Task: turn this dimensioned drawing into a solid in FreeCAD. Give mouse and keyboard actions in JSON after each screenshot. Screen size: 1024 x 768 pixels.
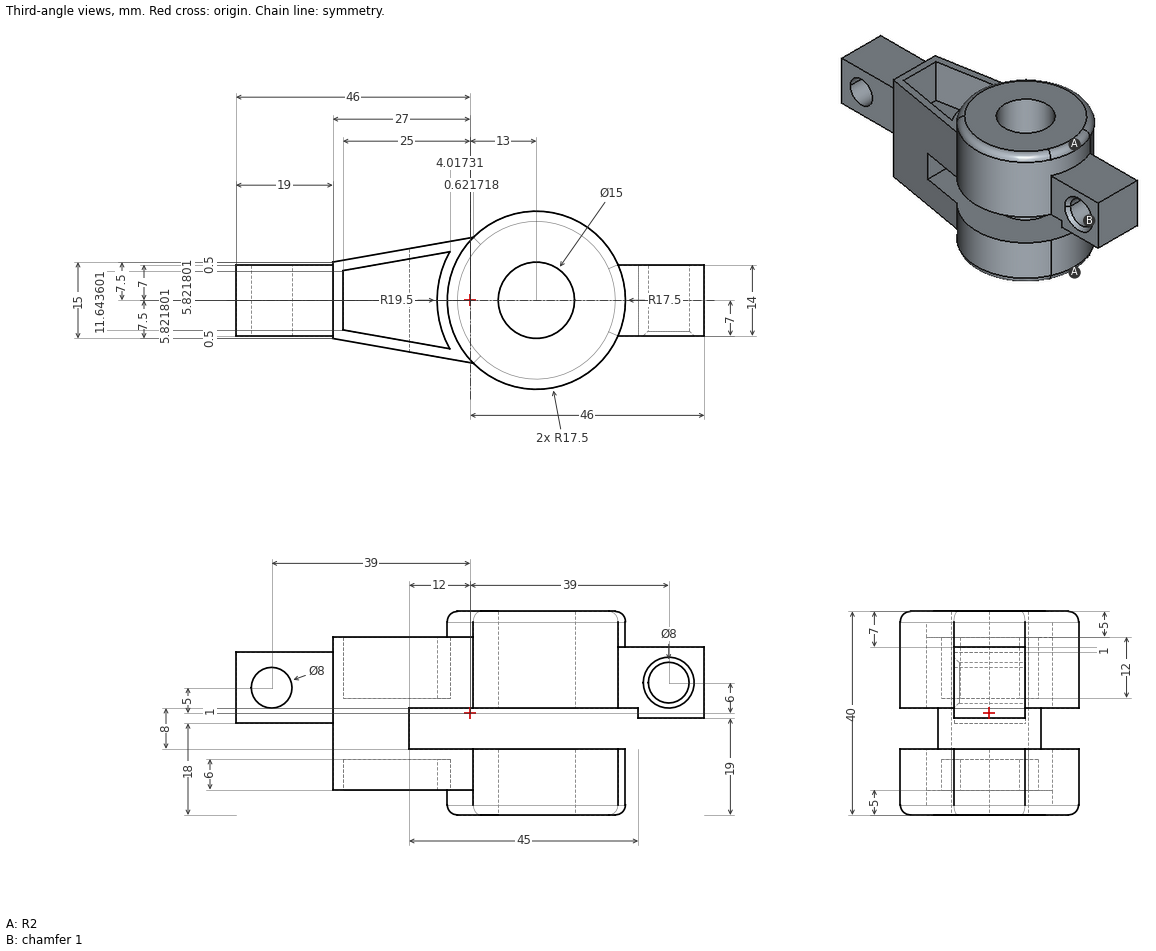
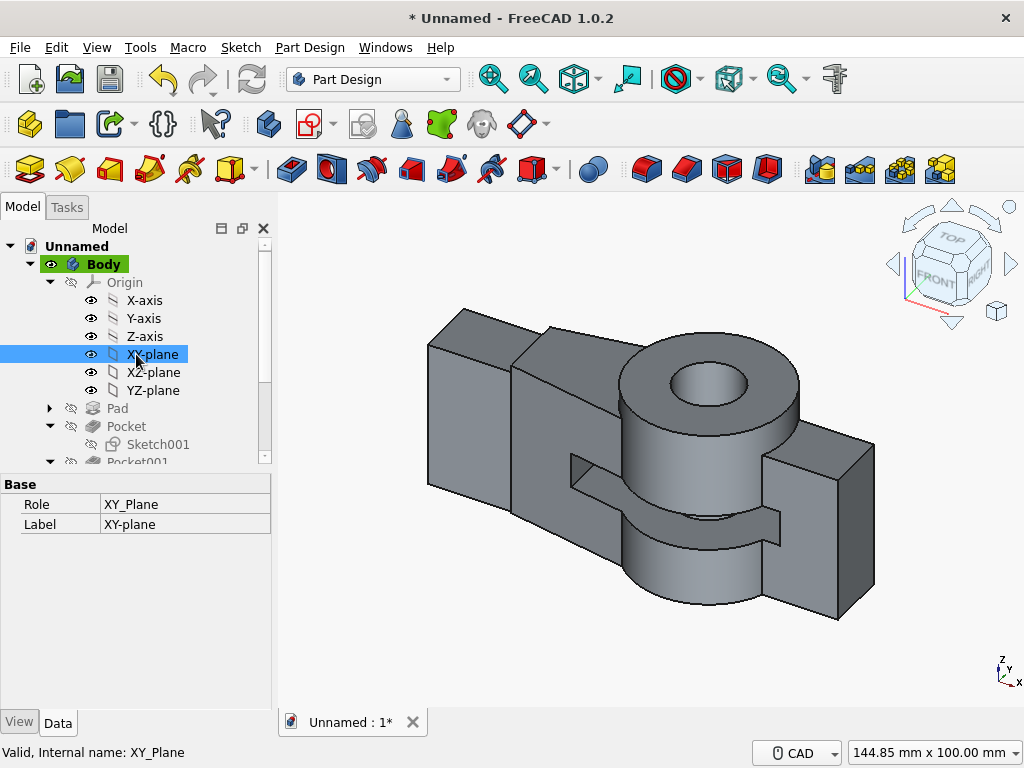
{"action": "left_click", "coordinate": [522, 124]}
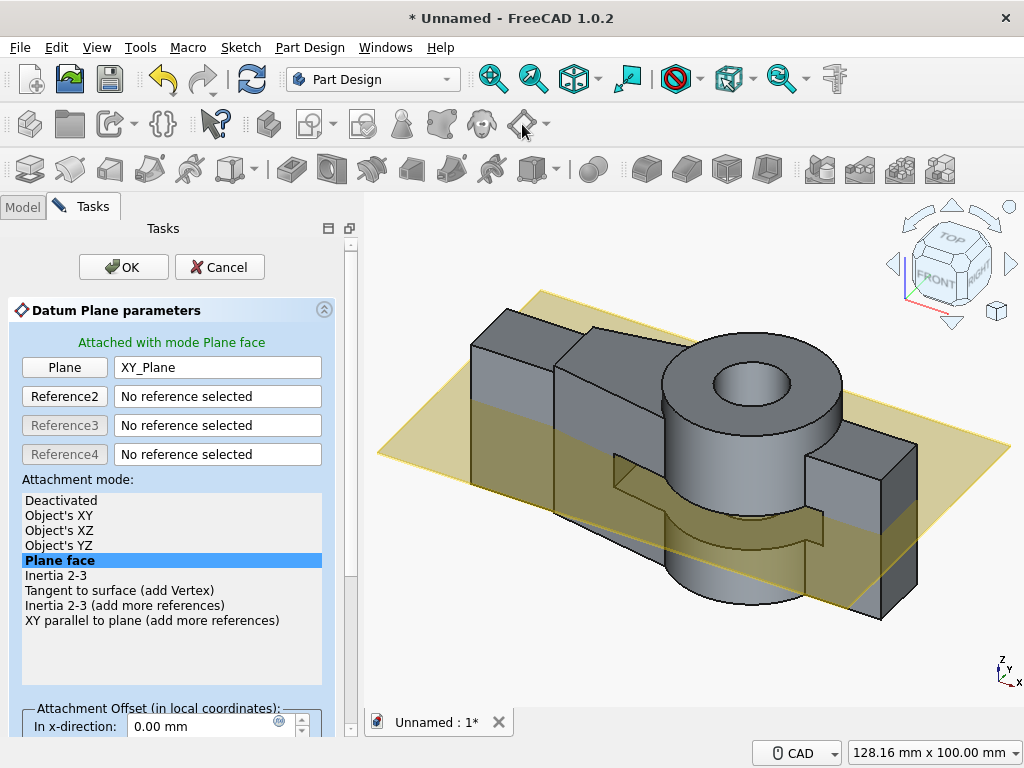
{"action": "scroll", "coordinate": [351, 487], "scroll_direction": "down", "scroll_amount": 3}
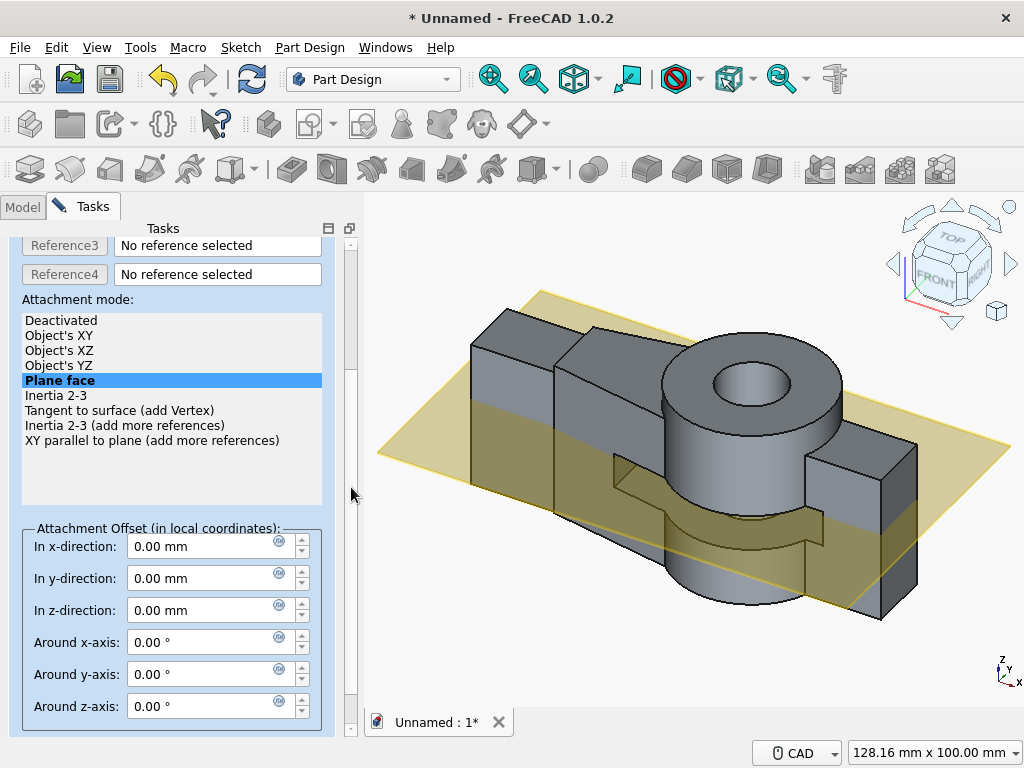
{"action": "triple_click", "coordinate": [210, 610]}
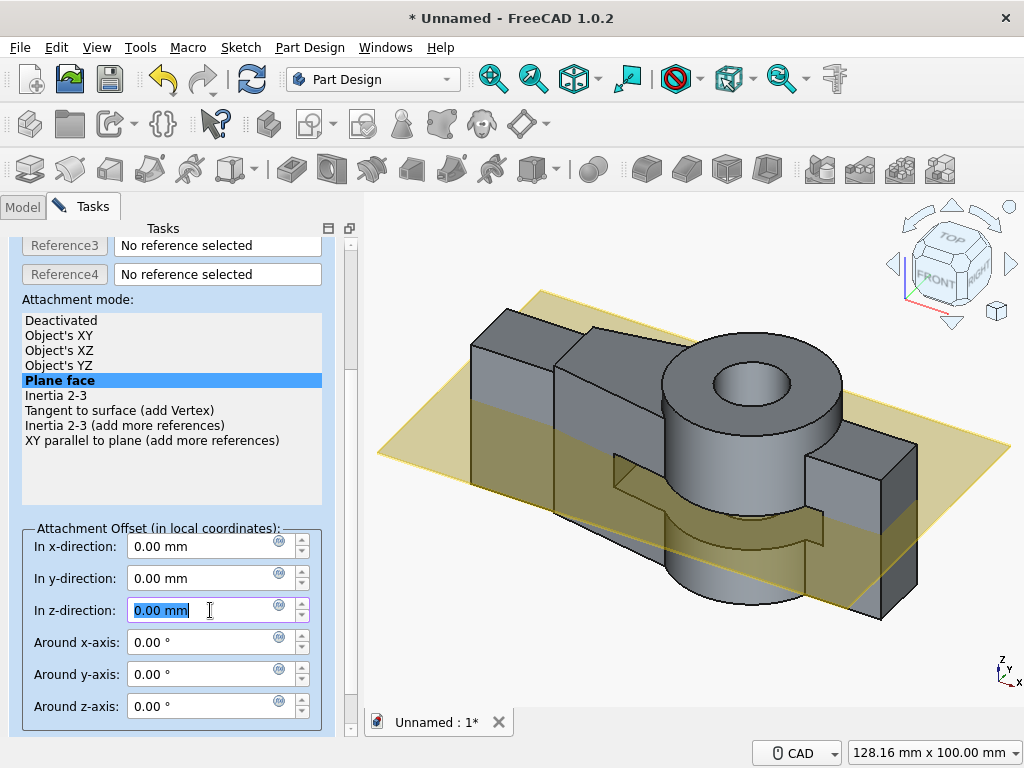
{"action": "type", "text": "-15"}
{"action": "key", "text": "Tab"}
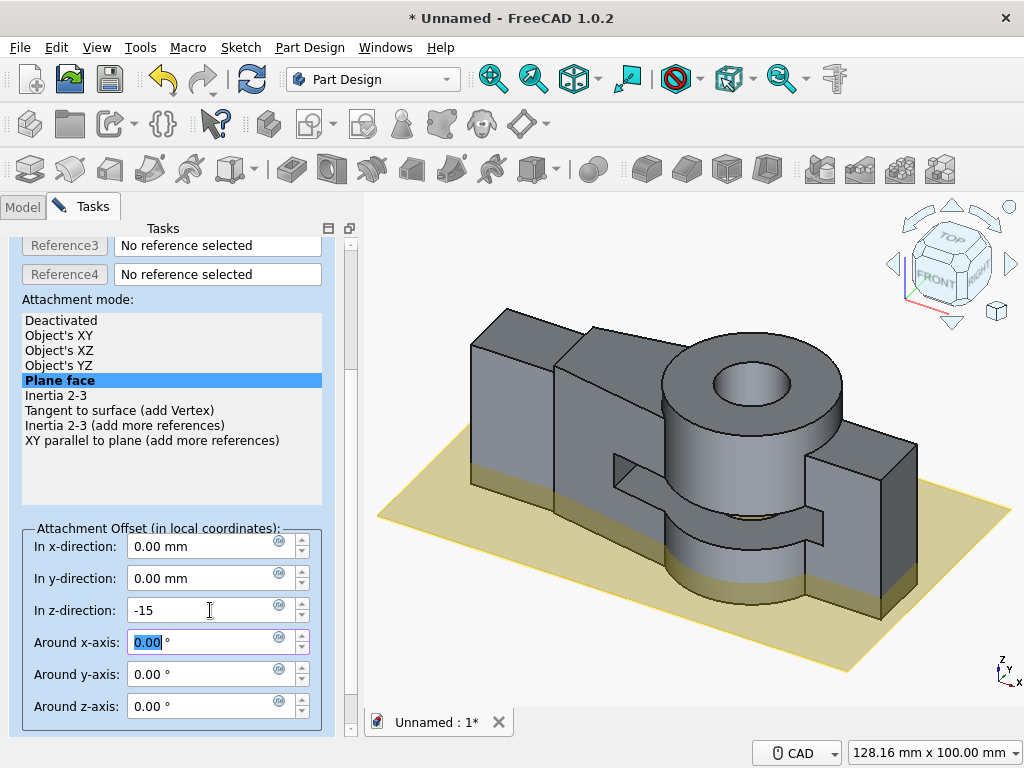
{"action": "scroll", "coordinate": [351, 487], "scroll_direction": "up", "scroll_amount": 4}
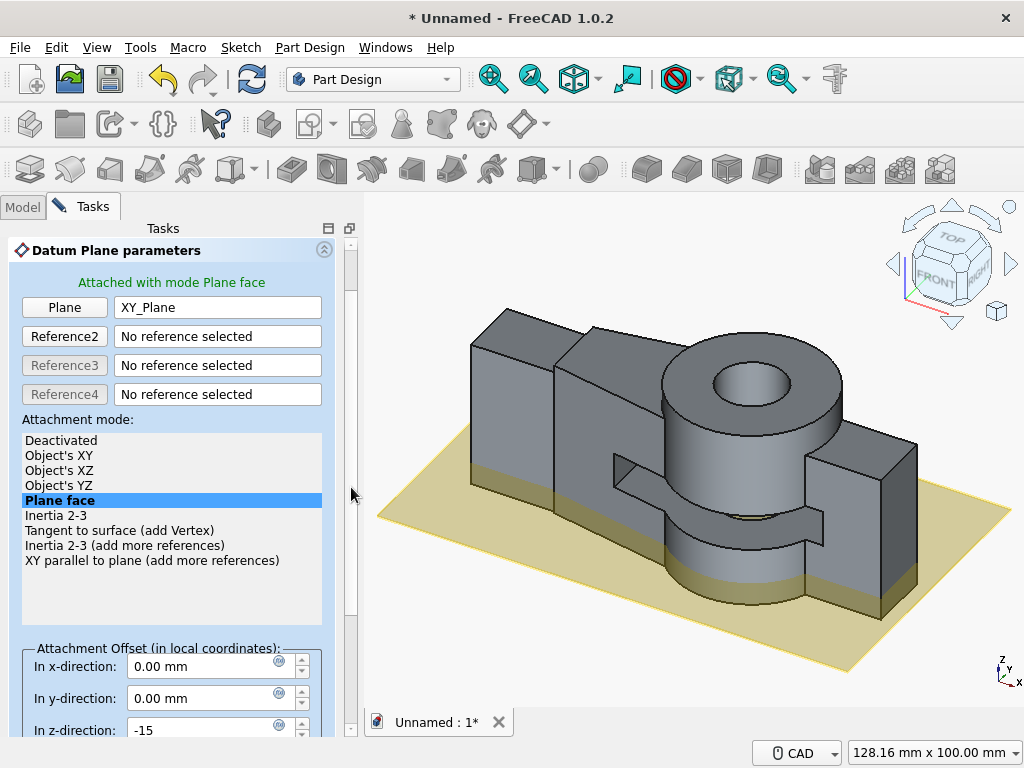
{"action": "left_click", "coordinate": [124, 267]}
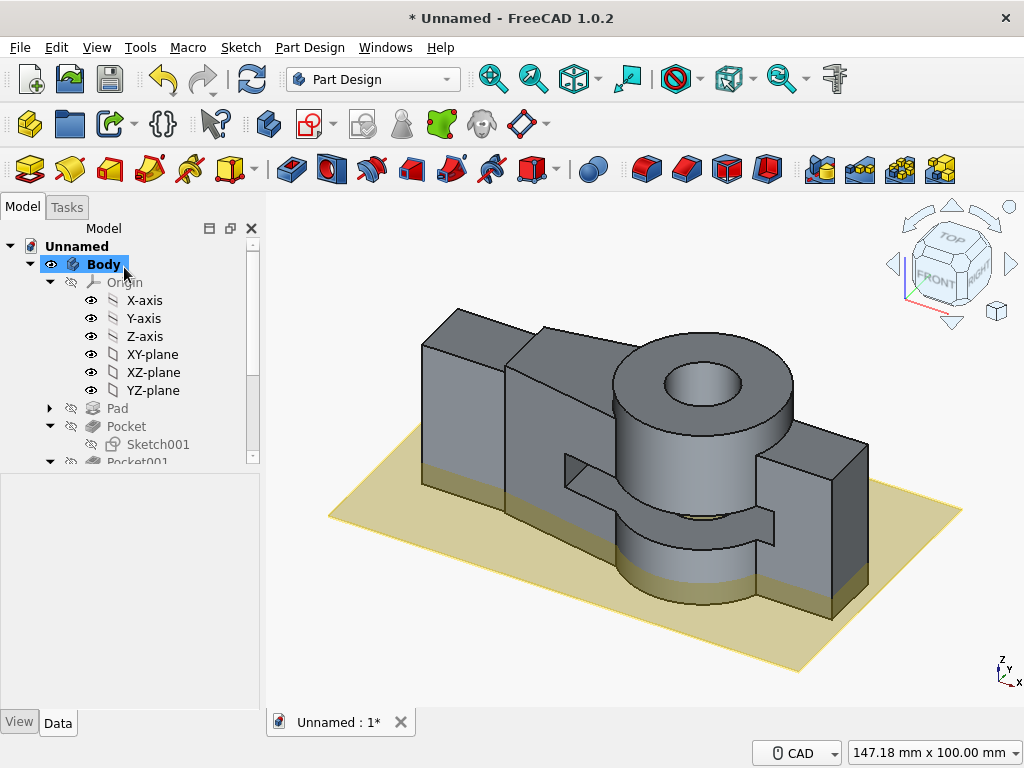
{"action": "scroll", "coordinate": [100, 350], "scroll_direction": "down", "scroll_amount": 3}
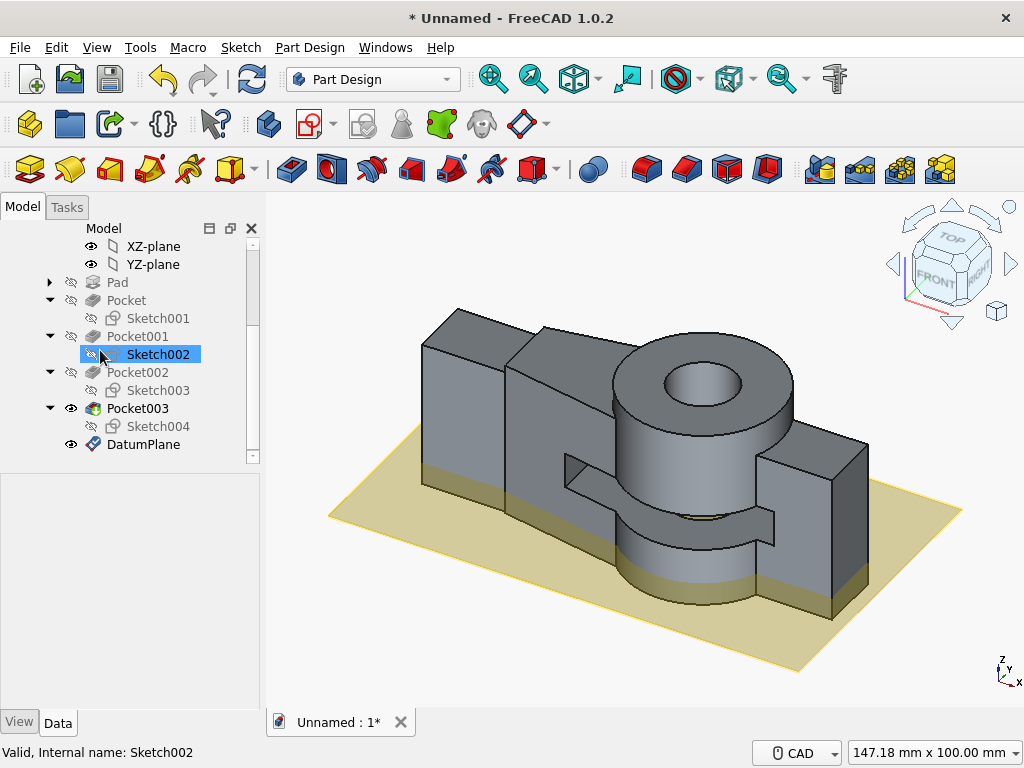
{"action": "left_click", "coordinate": [116, 444]}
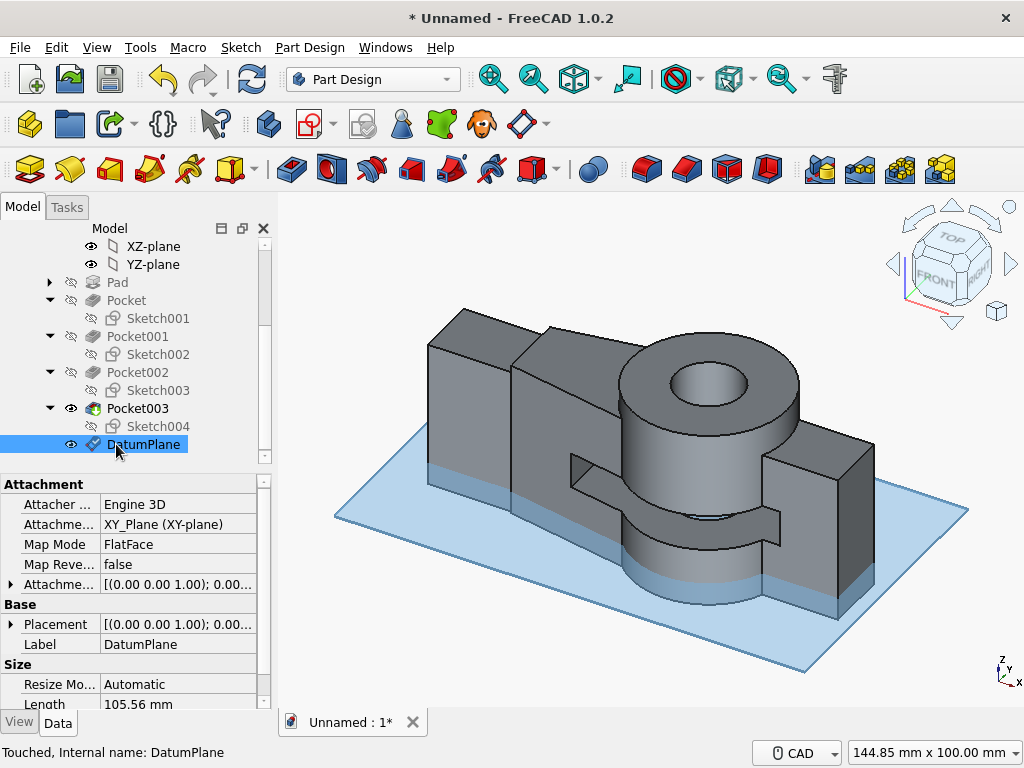
{"action": "left_click", "coordinate": [310, 124]}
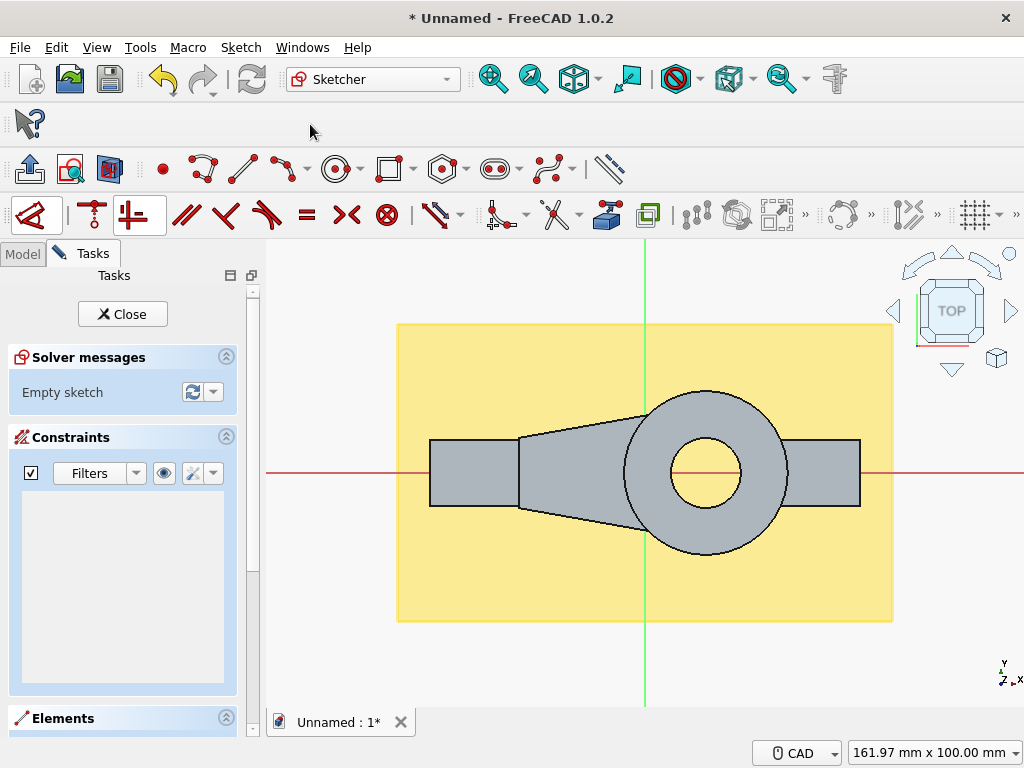
{"action": "left_click", "coordinate": [110, 170]}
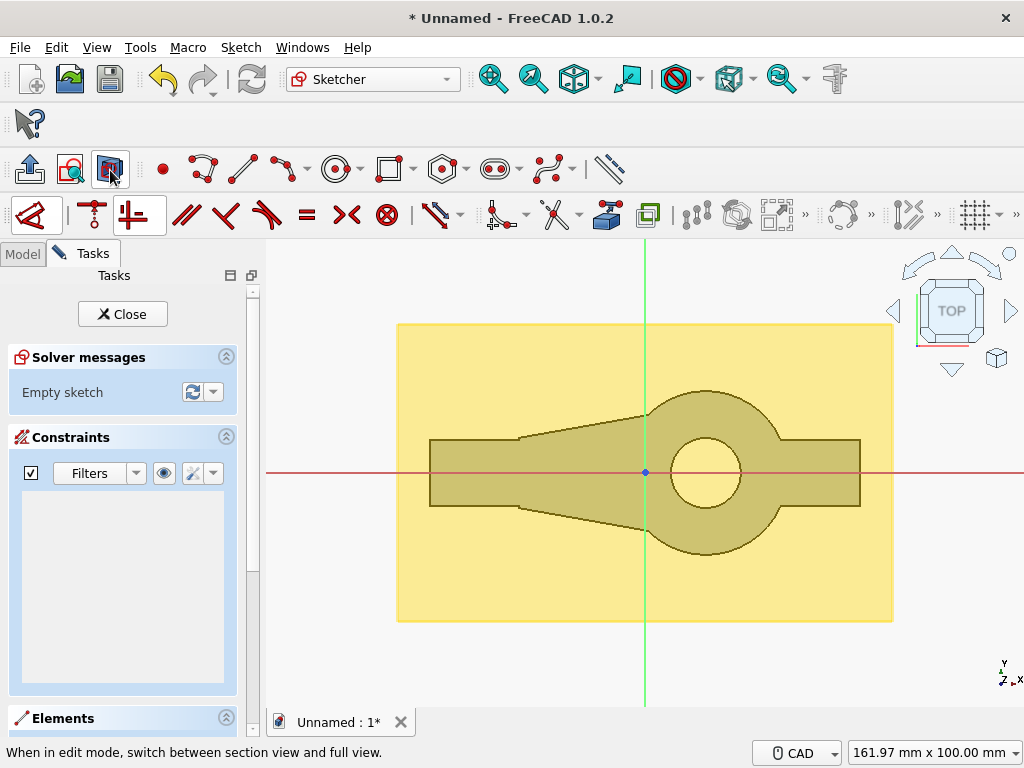
{"action": "scroll", "coordinate": [587, 473], "scroll_direction": "up", "scroll_amount": 5}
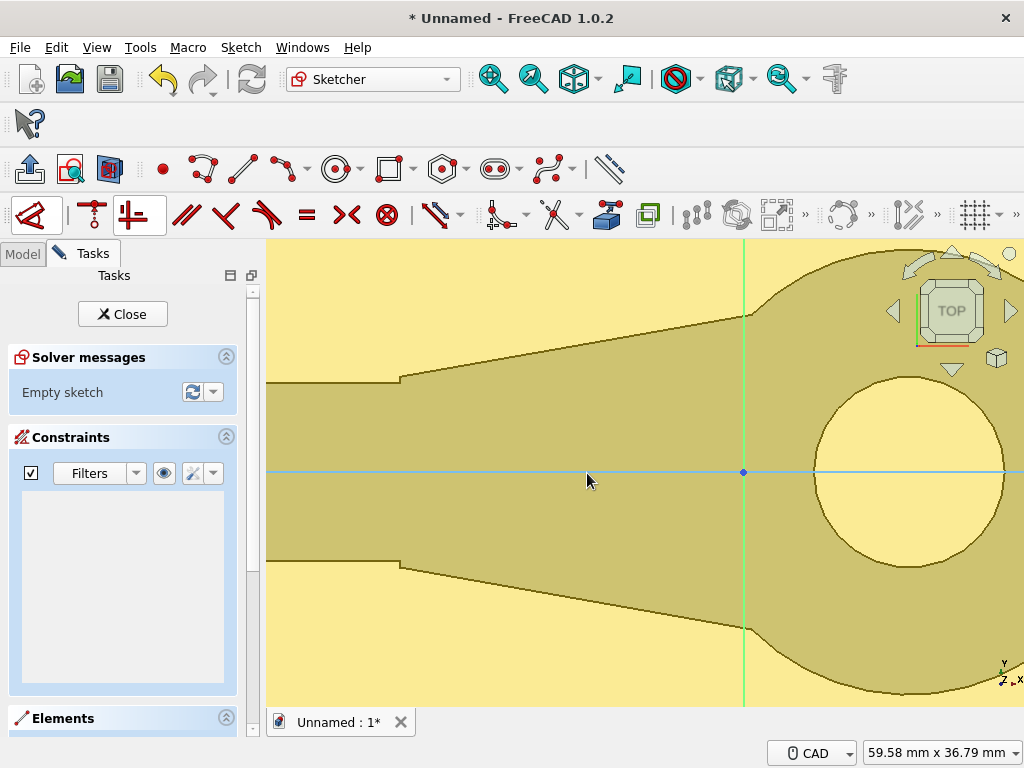
{"action": "left_click", "coordinate": [204, 170]}